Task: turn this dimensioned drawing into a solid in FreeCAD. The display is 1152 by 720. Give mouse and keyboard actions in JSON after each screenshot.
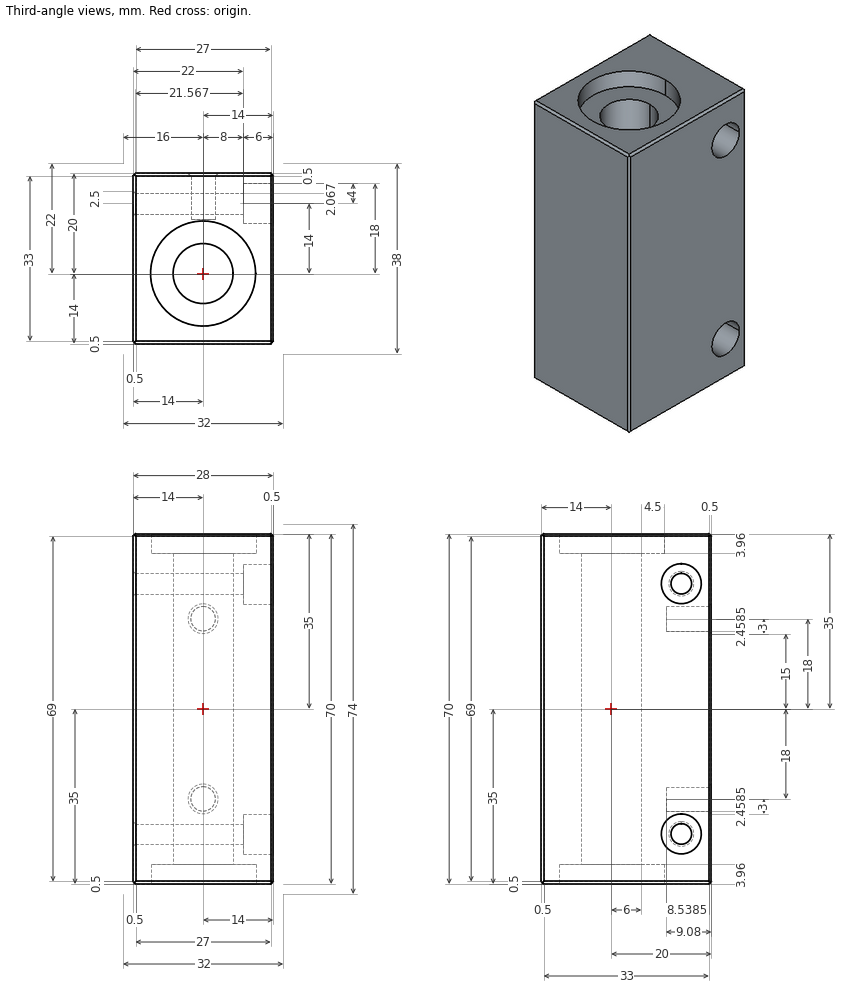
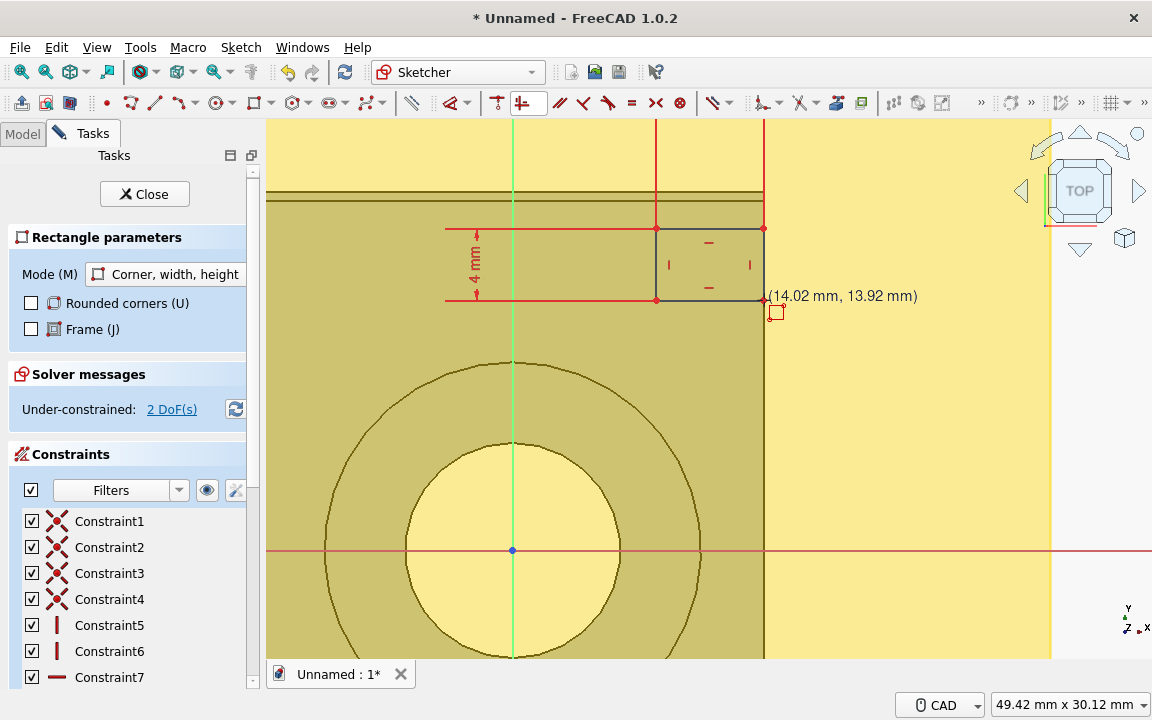
{"action": "left_click", "coordinate": [156, 104]}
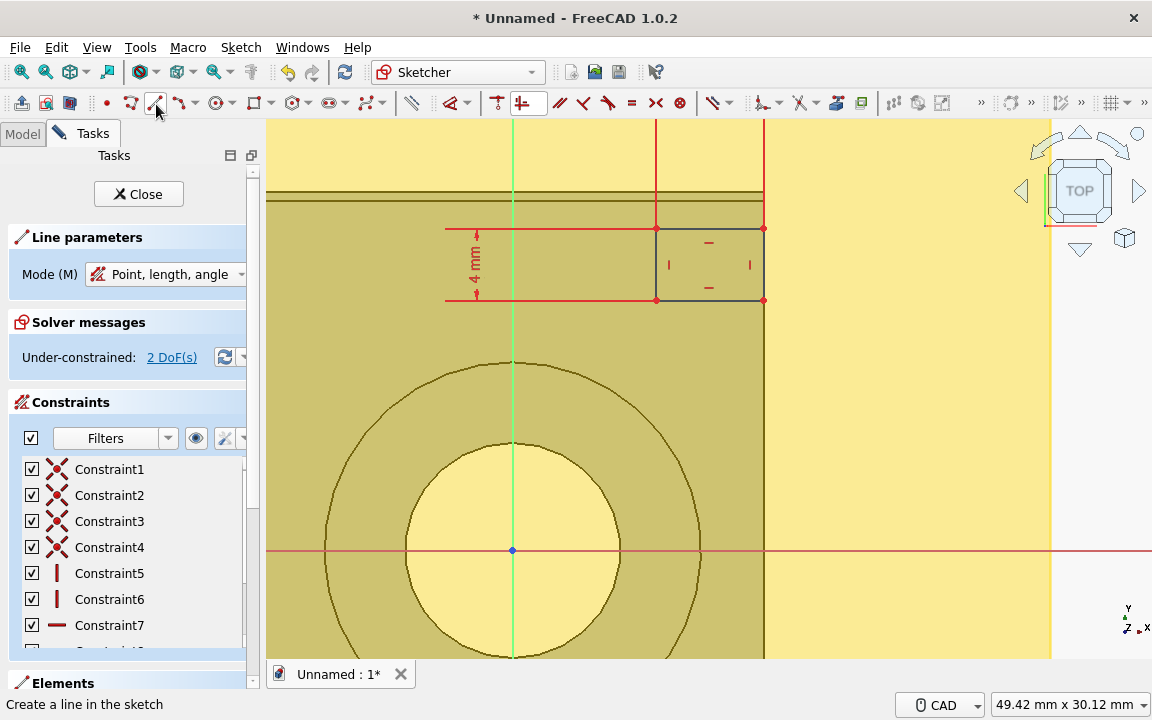
{"action": "scroll", "coordinate": [645, 300], "scroll_direction": "up", "scroll_amount": 2}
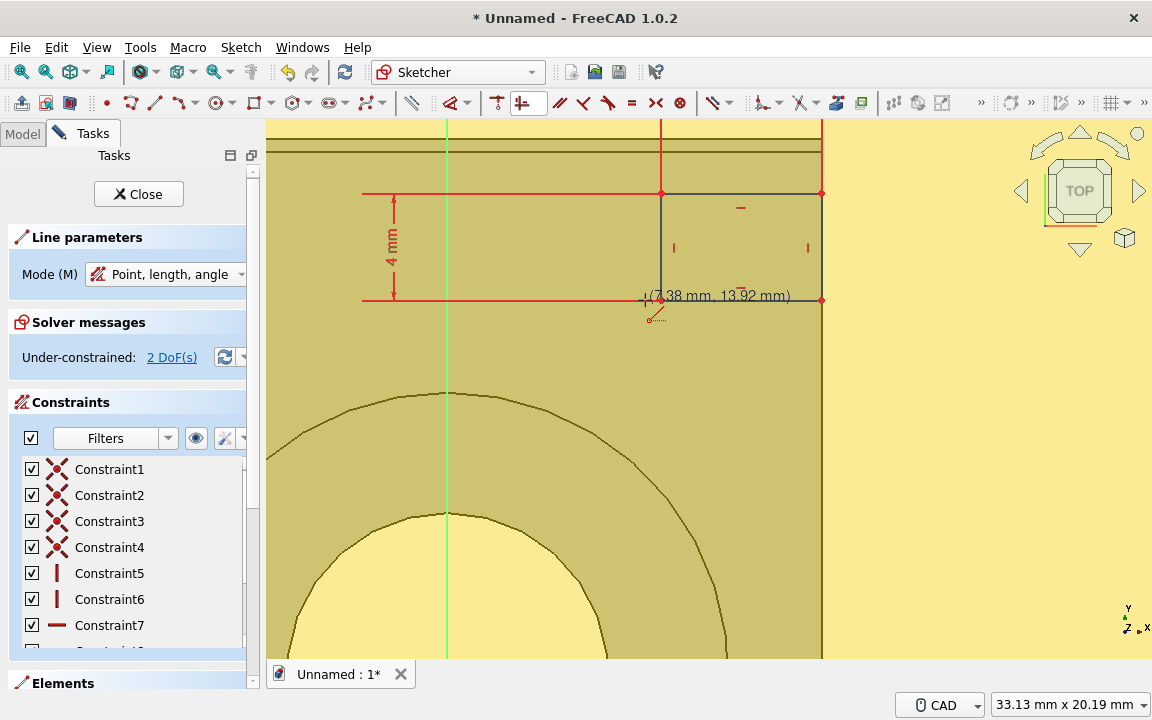
{"action": "left_click", "coordinate": [645, 299]}
{"action": "left_click", "coordinate": [597, 299]}
{"action": "key", "text": "Escape"}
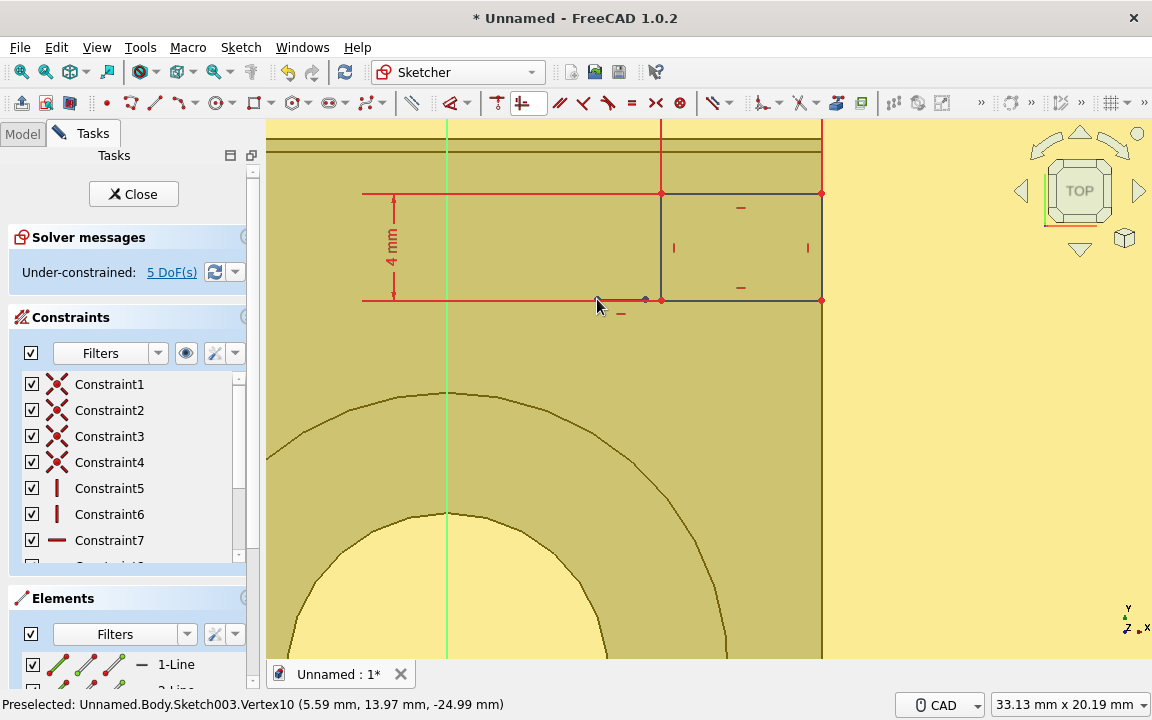
{"action": "left_click", "coordinate": [631, 300]}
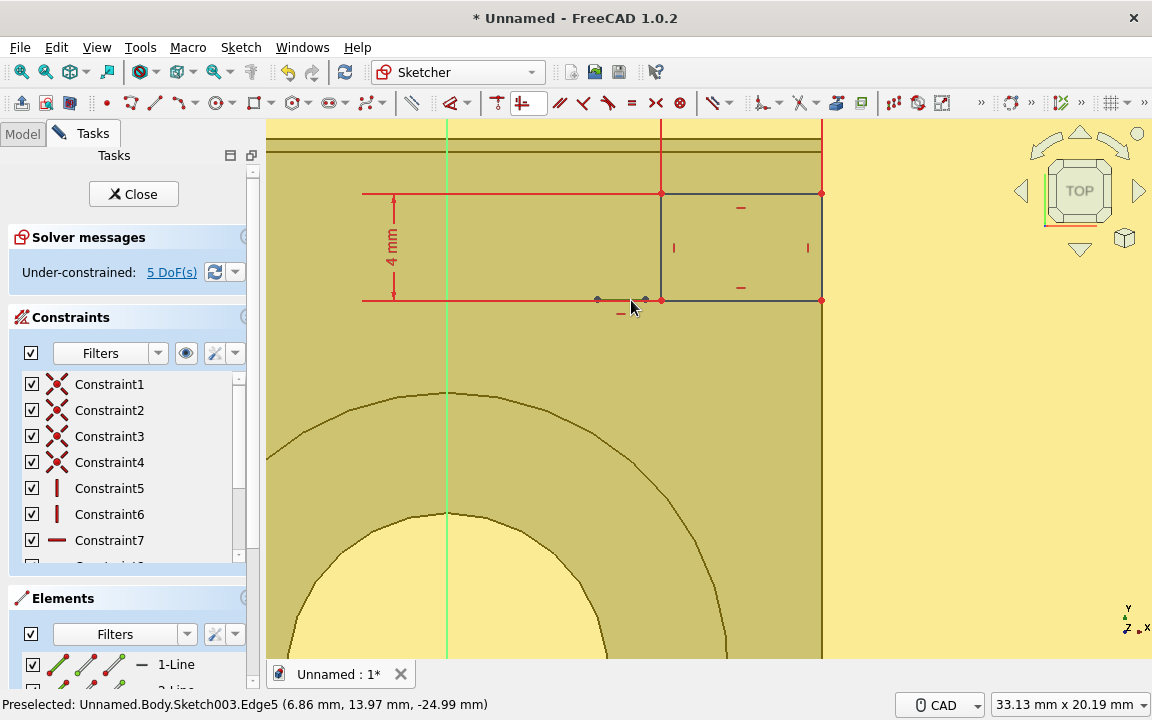
{"action": "left_click", "coordinate": [412, 104]}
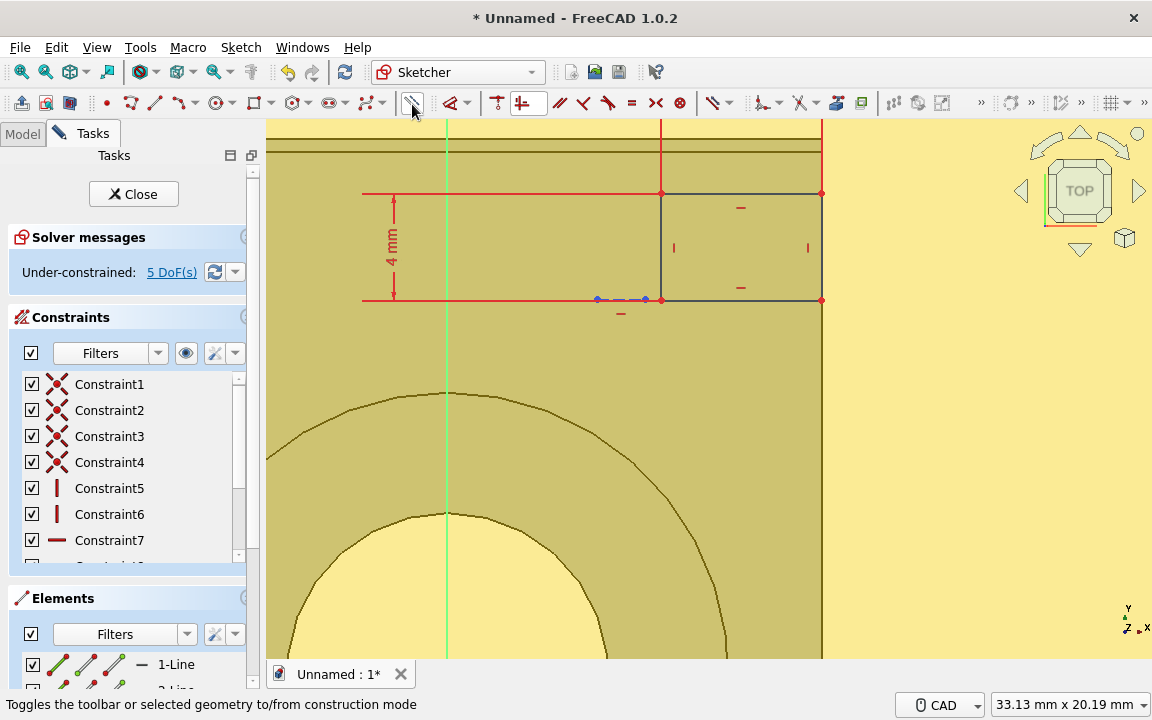
{"action": "left_click", "coordinate": [450, 104]}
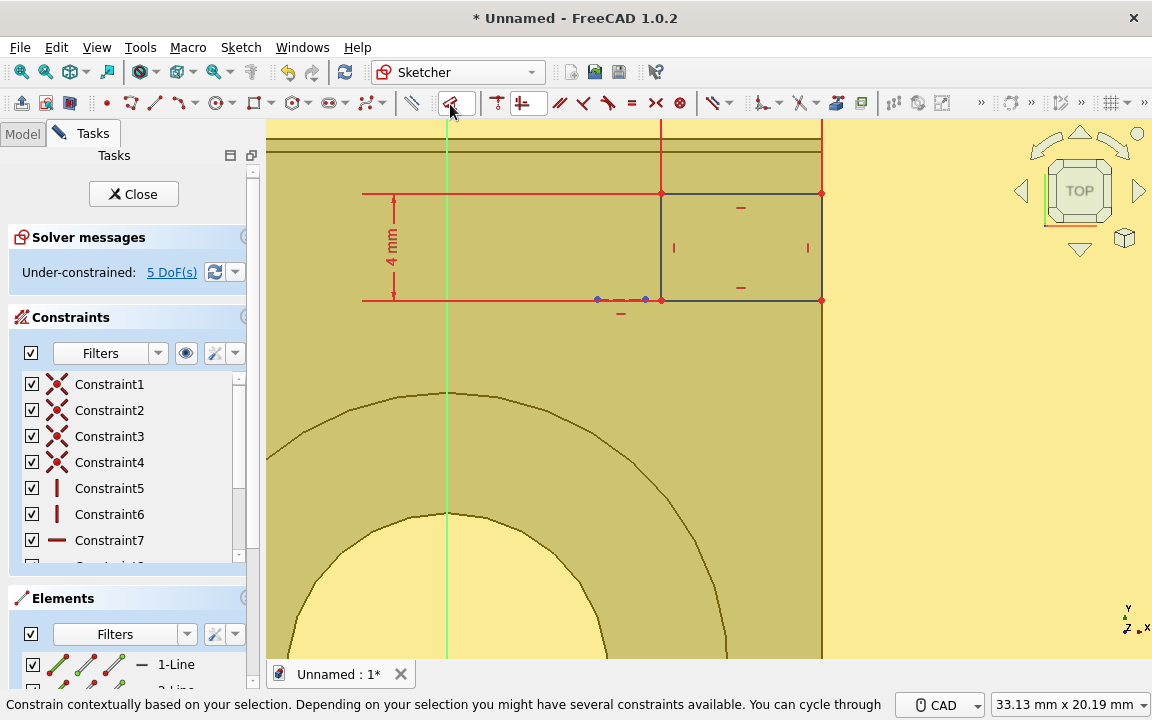
{"action": "left_click", "coordinate": [661, 194]}
{"action": "left_click", "coordinate": [554, 160]}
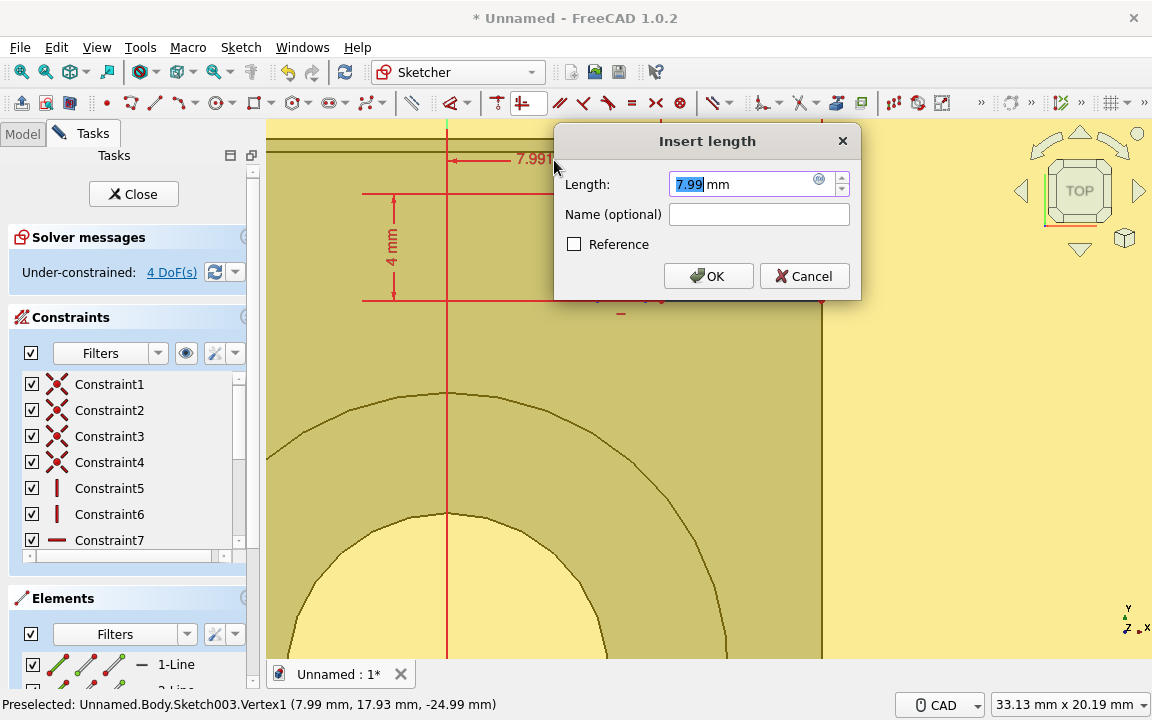
{"action": "type", "text": "8"}
{"action": "key", "text": "Return"}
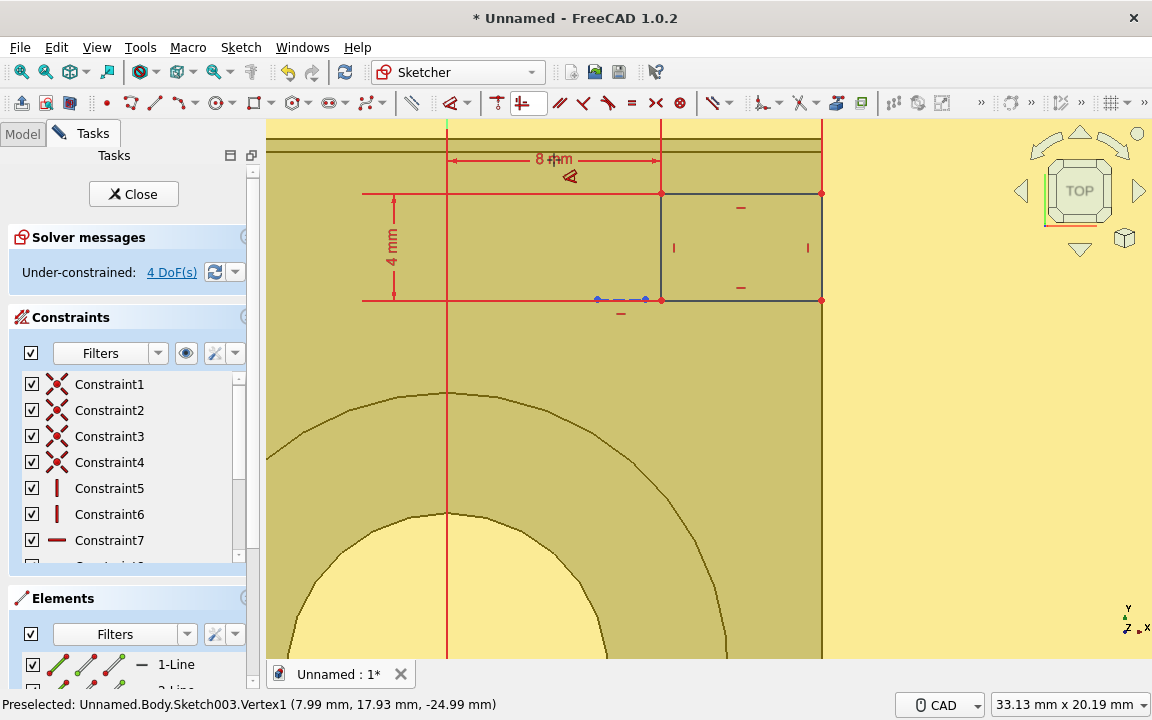
{"action": "left_click", "coordinate": [661, 194]}
{"action": "left_click", "coordinate": [413, 412]}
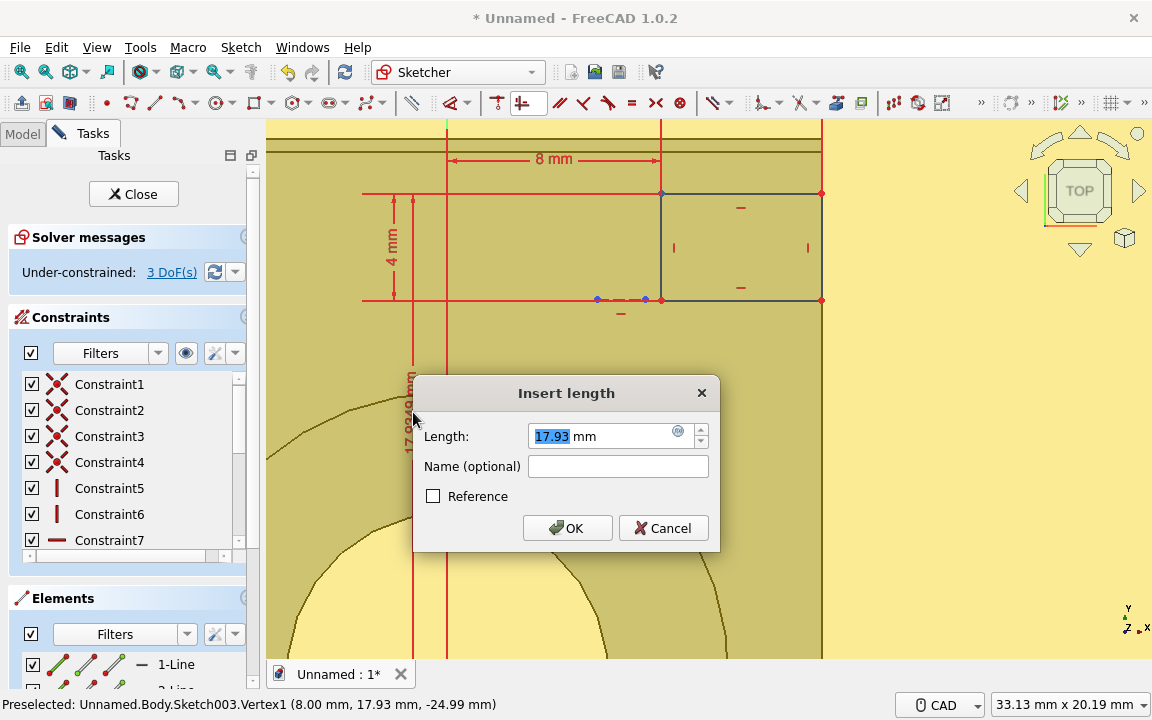
{"action": "type", "text": "18"}
{"action": "key", "text": "Return"}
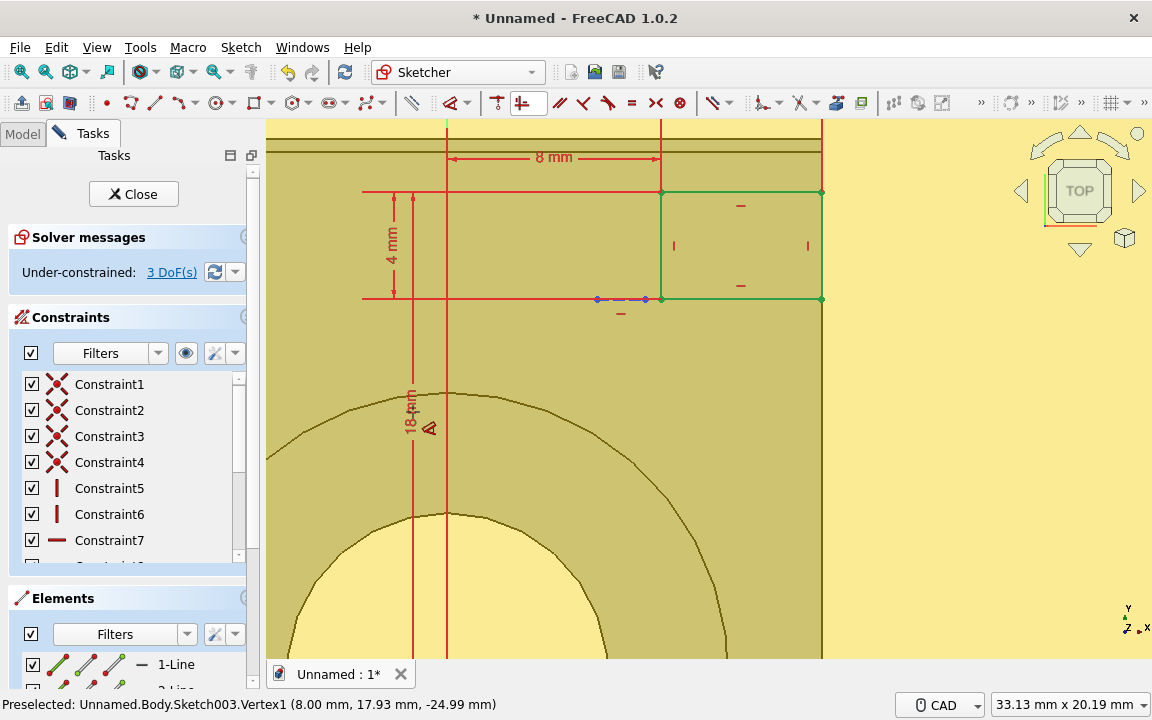
{"action": "left_click", "coordinate": [645, 300]}
{"action": "left_click", "coordinate": [413, 466]}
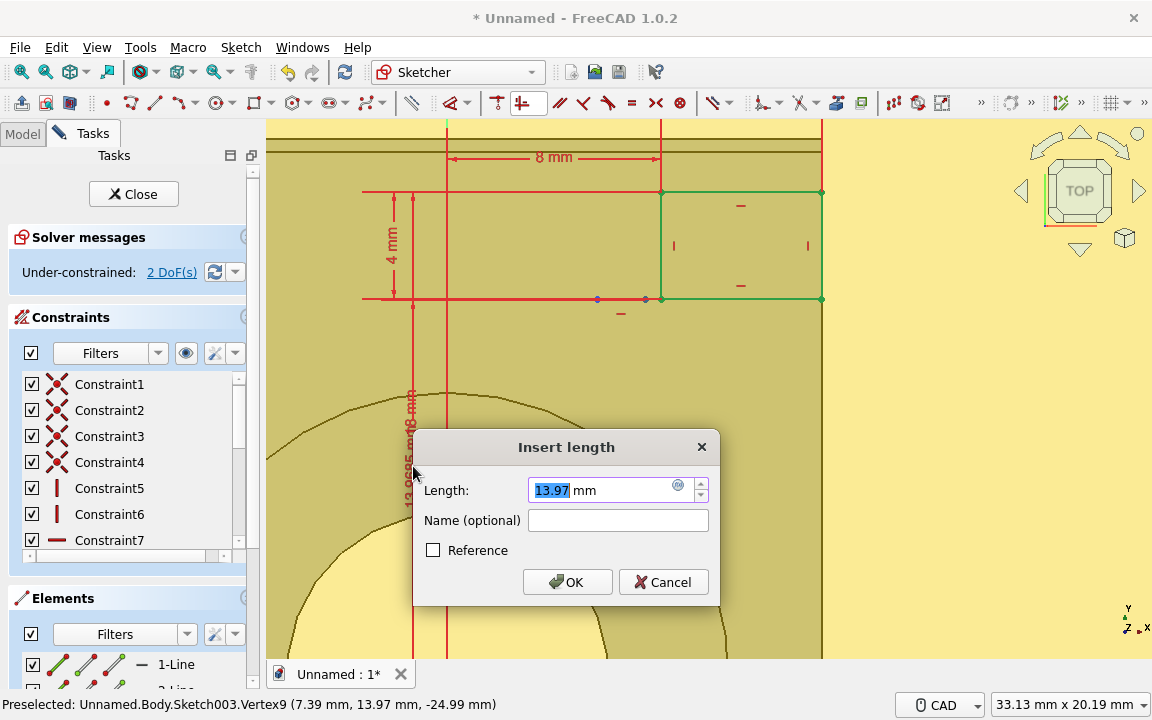
{"action": "type", "text": "14"}
{"action": "key", "text": "Return"}
{"action": "key", "text": "Escape"}